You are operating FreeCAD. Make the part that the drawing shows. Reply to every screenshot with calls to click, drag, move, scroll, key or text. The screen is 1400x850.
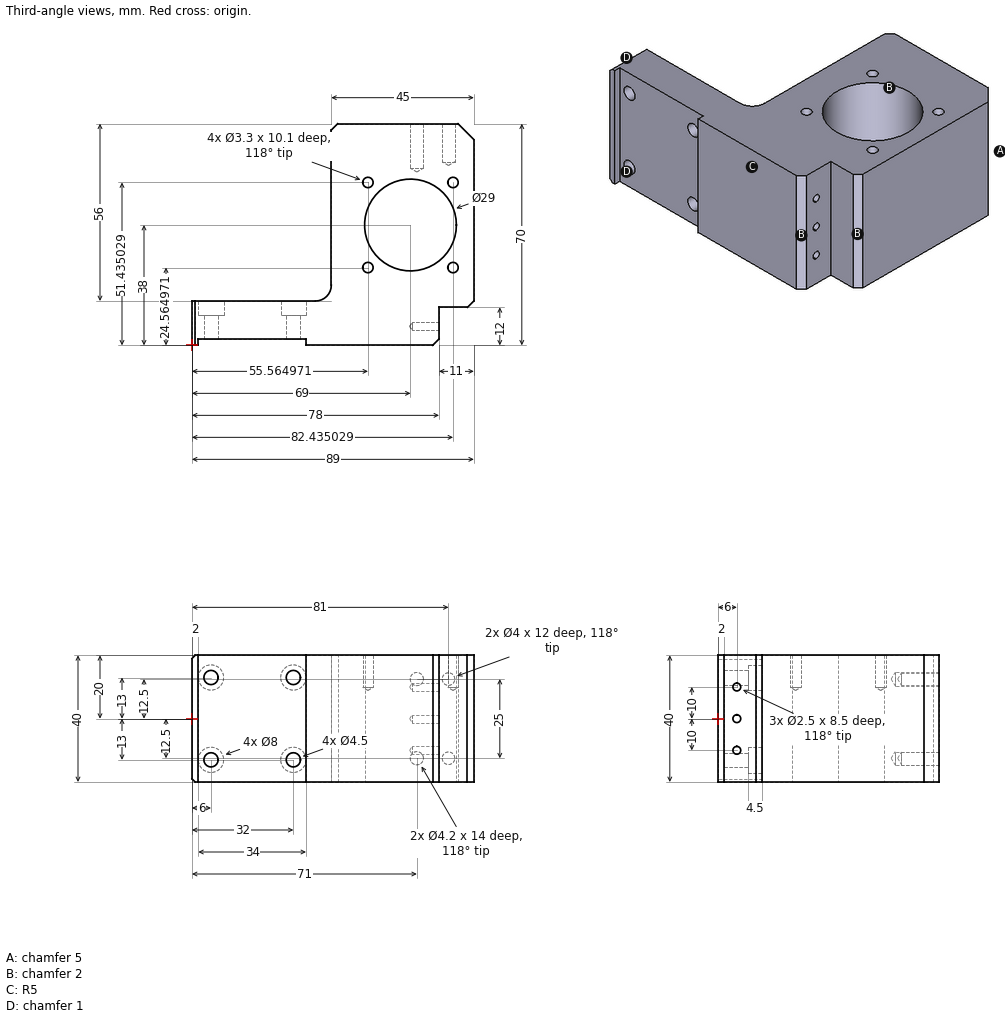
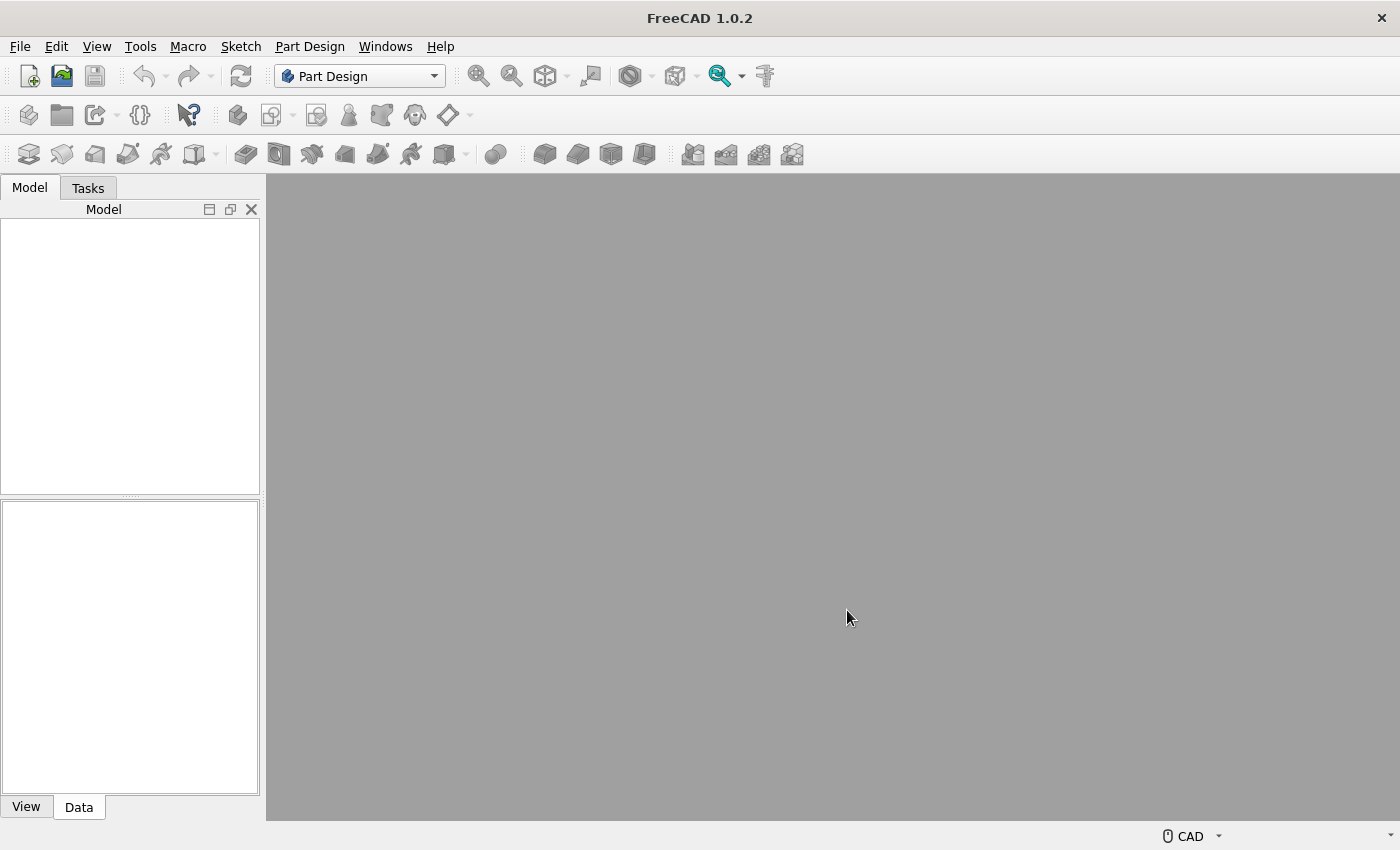
click(29, 76)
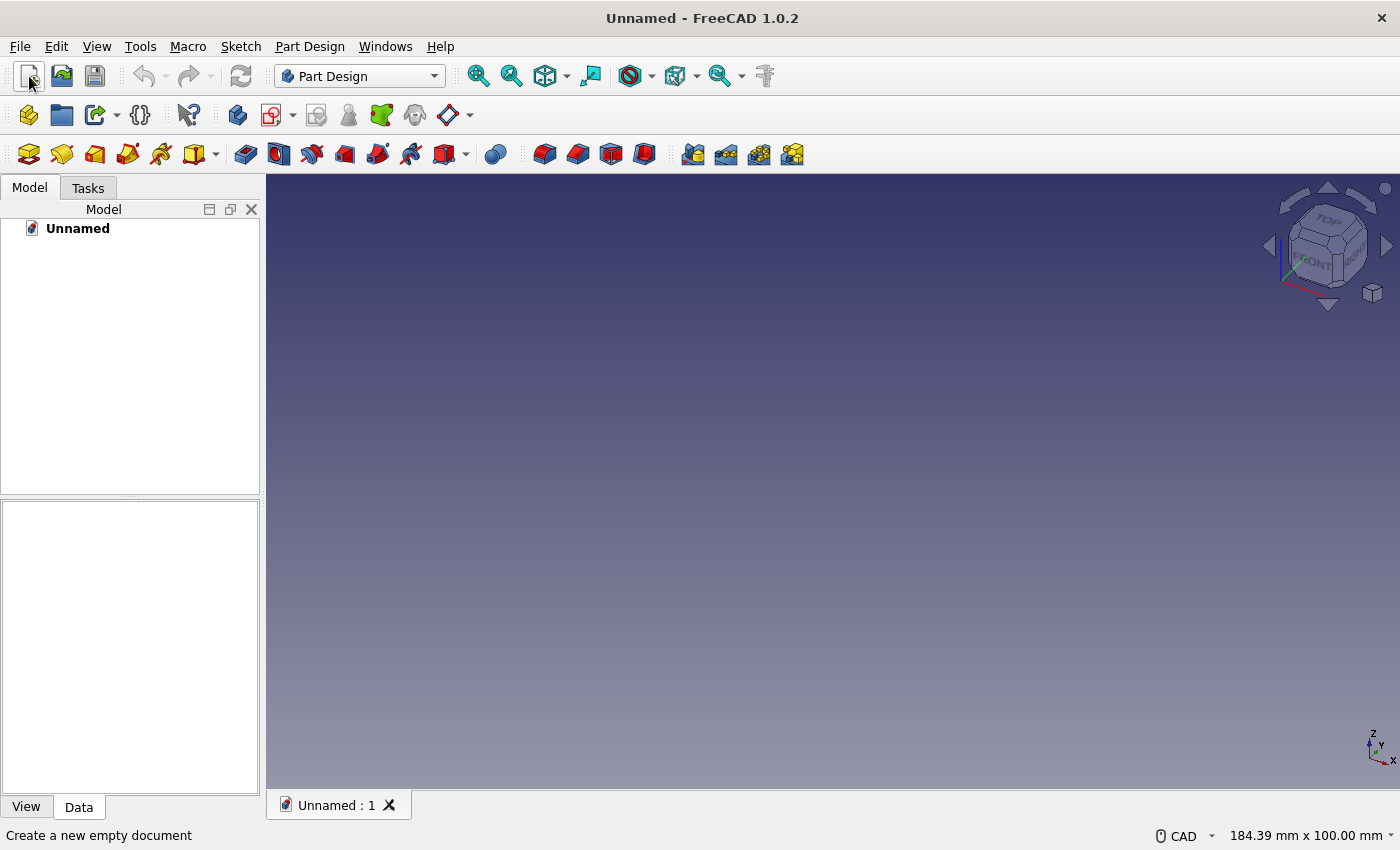
click(270, 116)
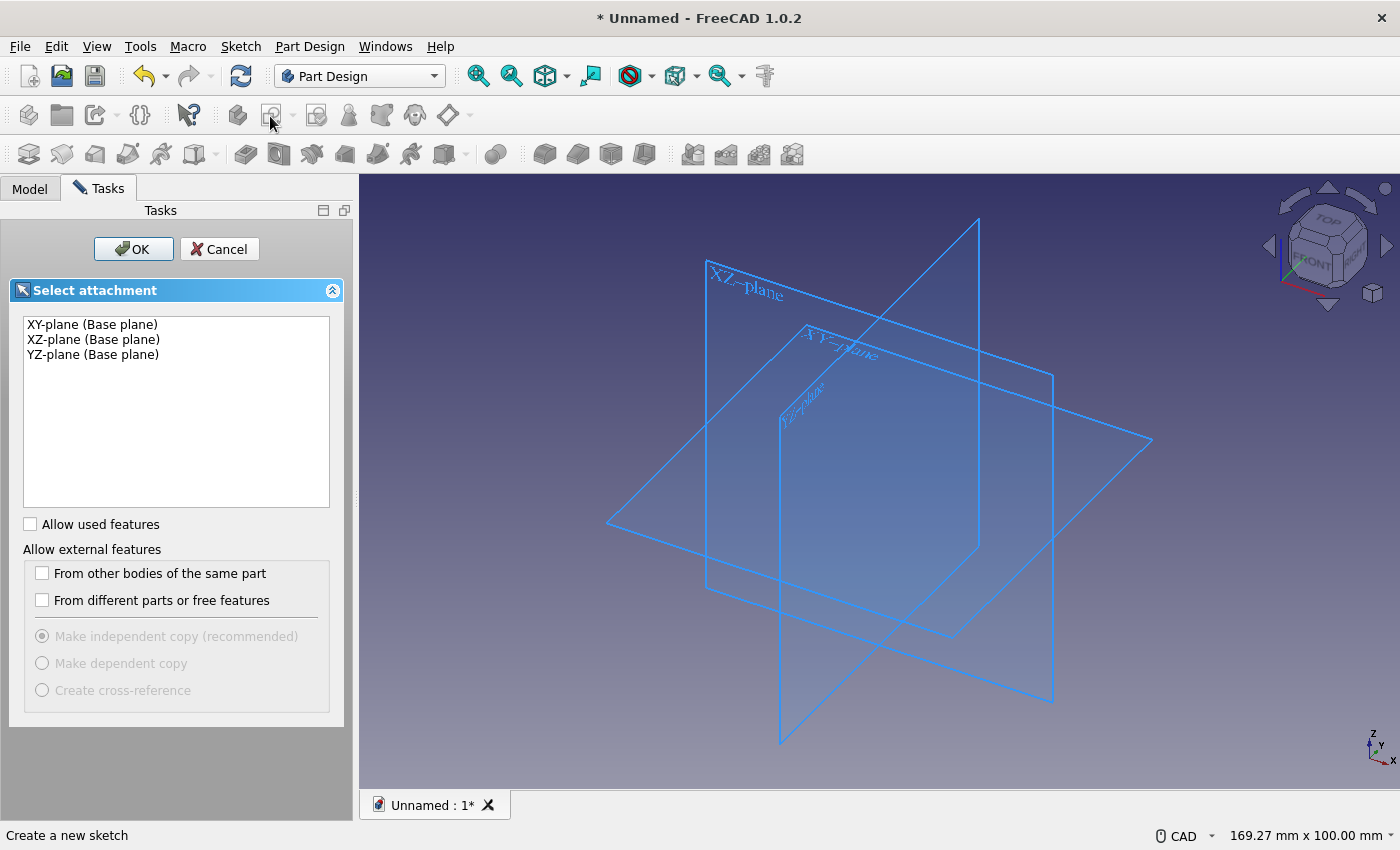
click(84, 324)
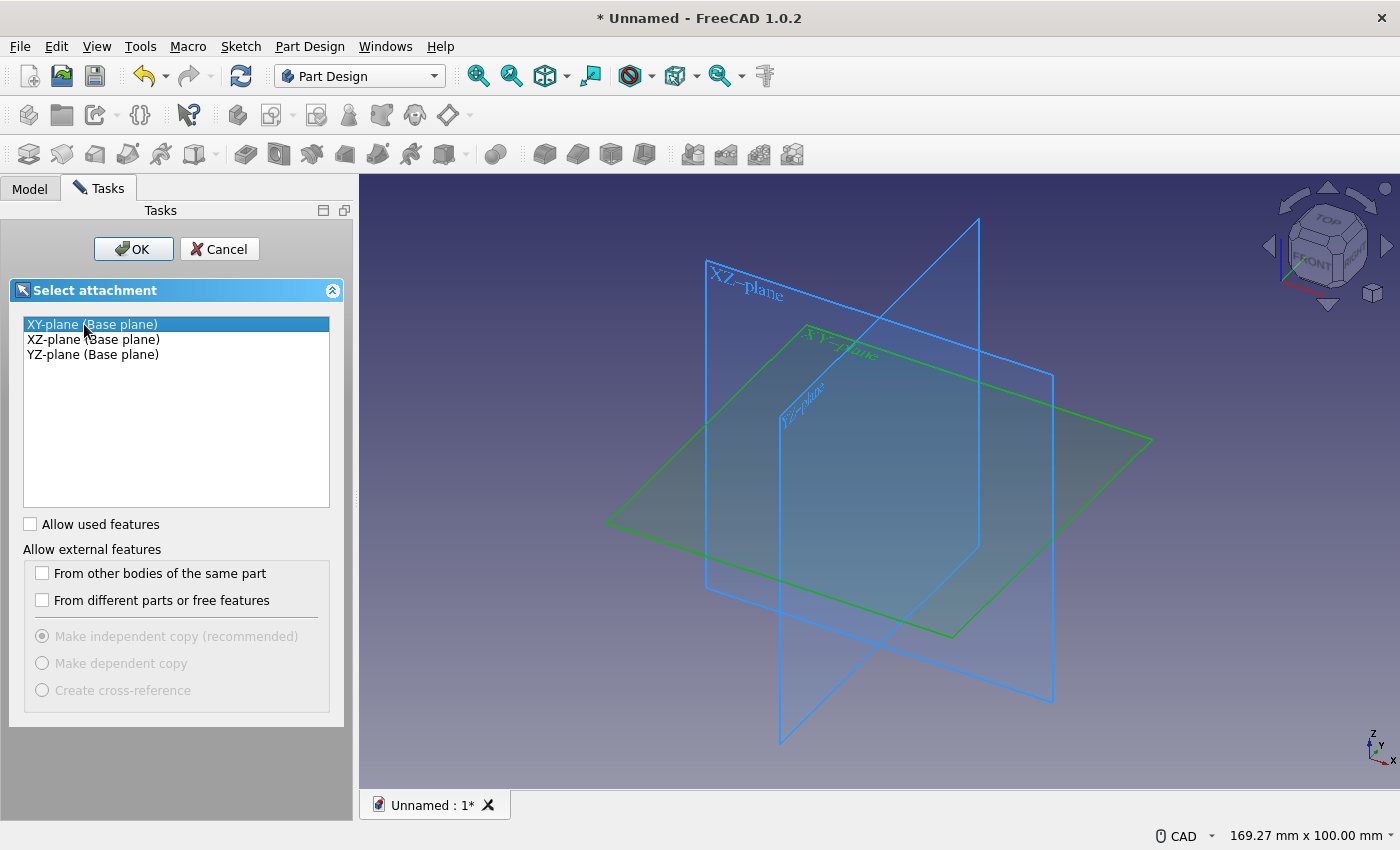
click(134, 249)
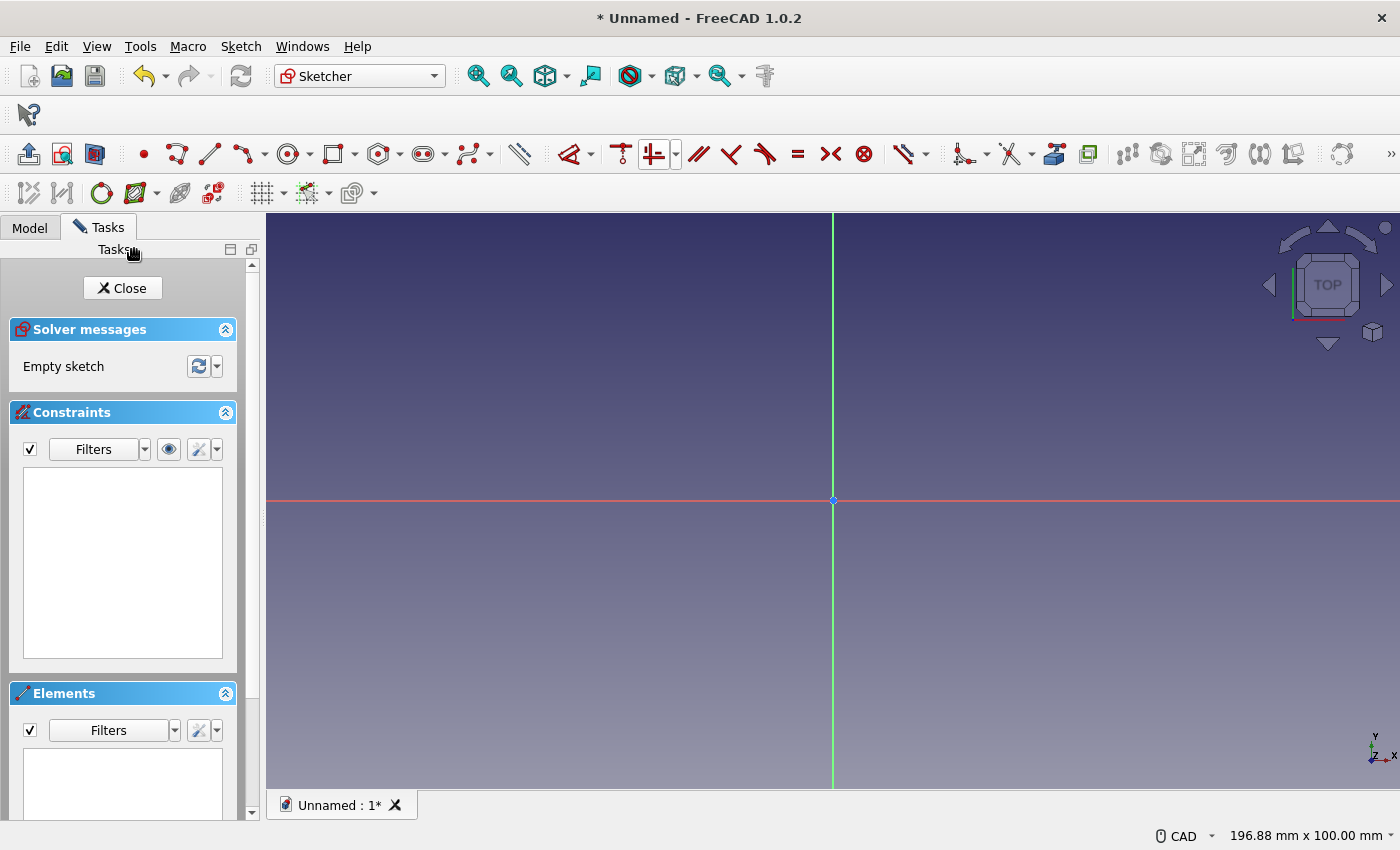
scroll(294, 761, down, 2)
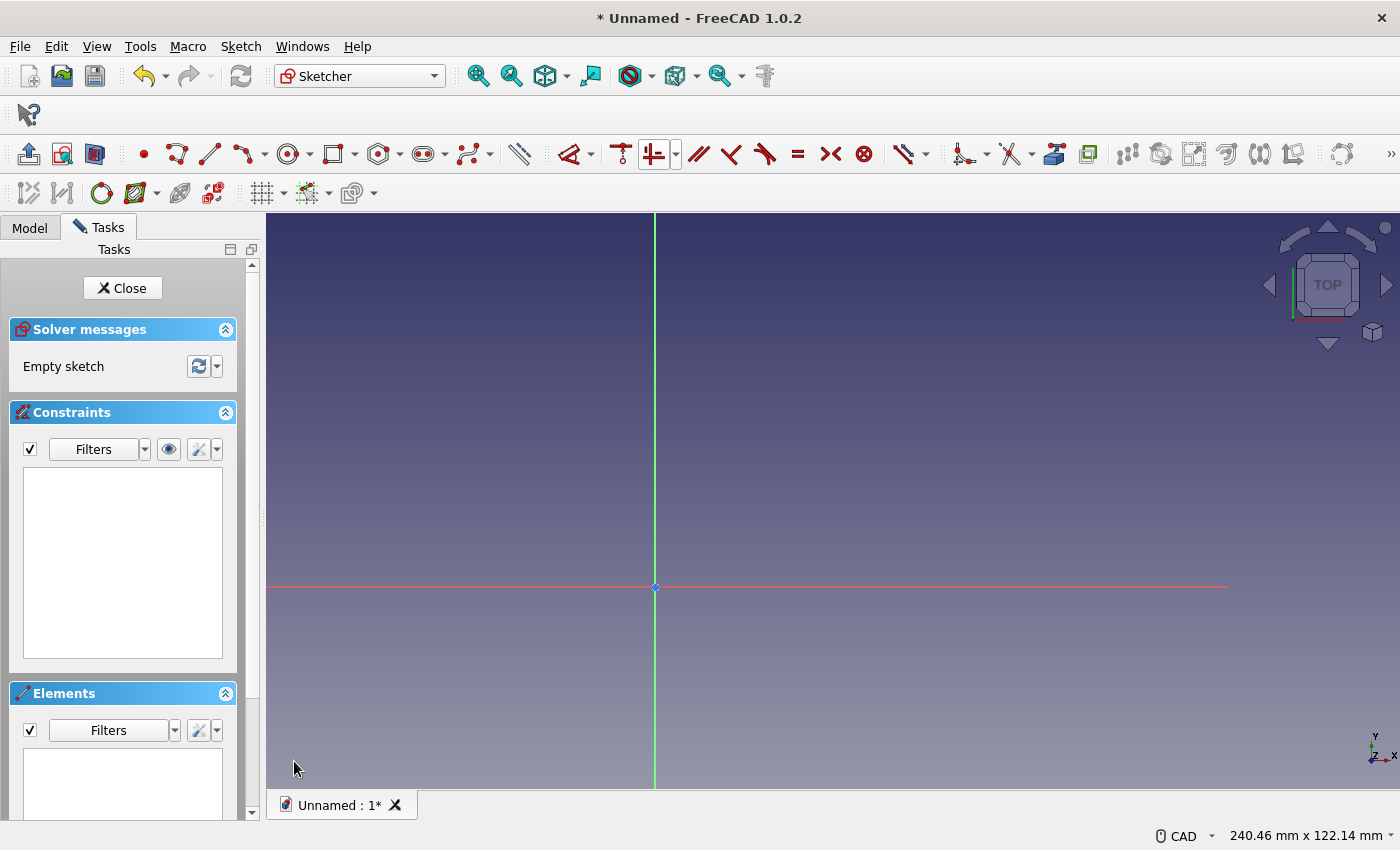
scroll(954, 352, up, 2)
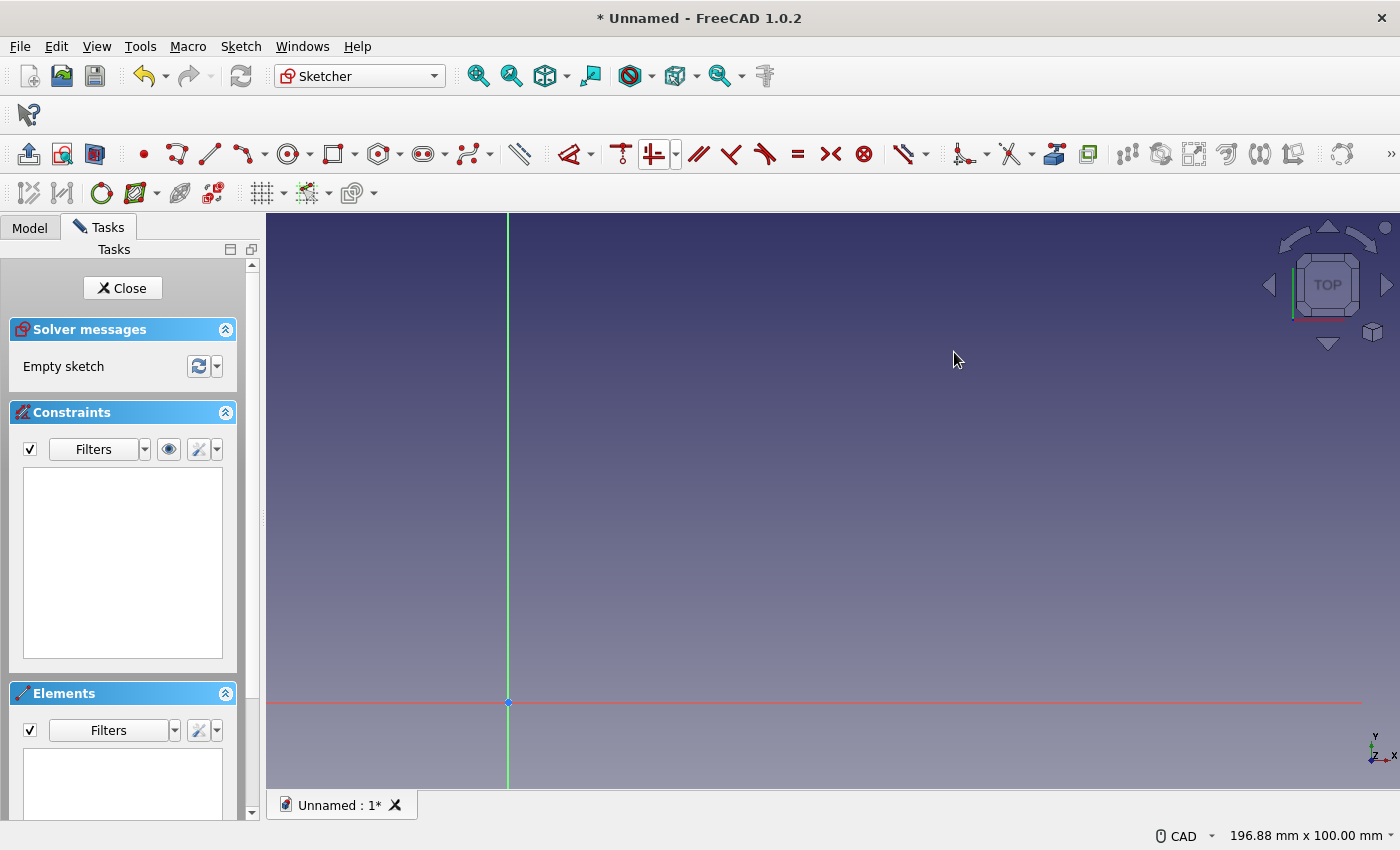
click(177, 154)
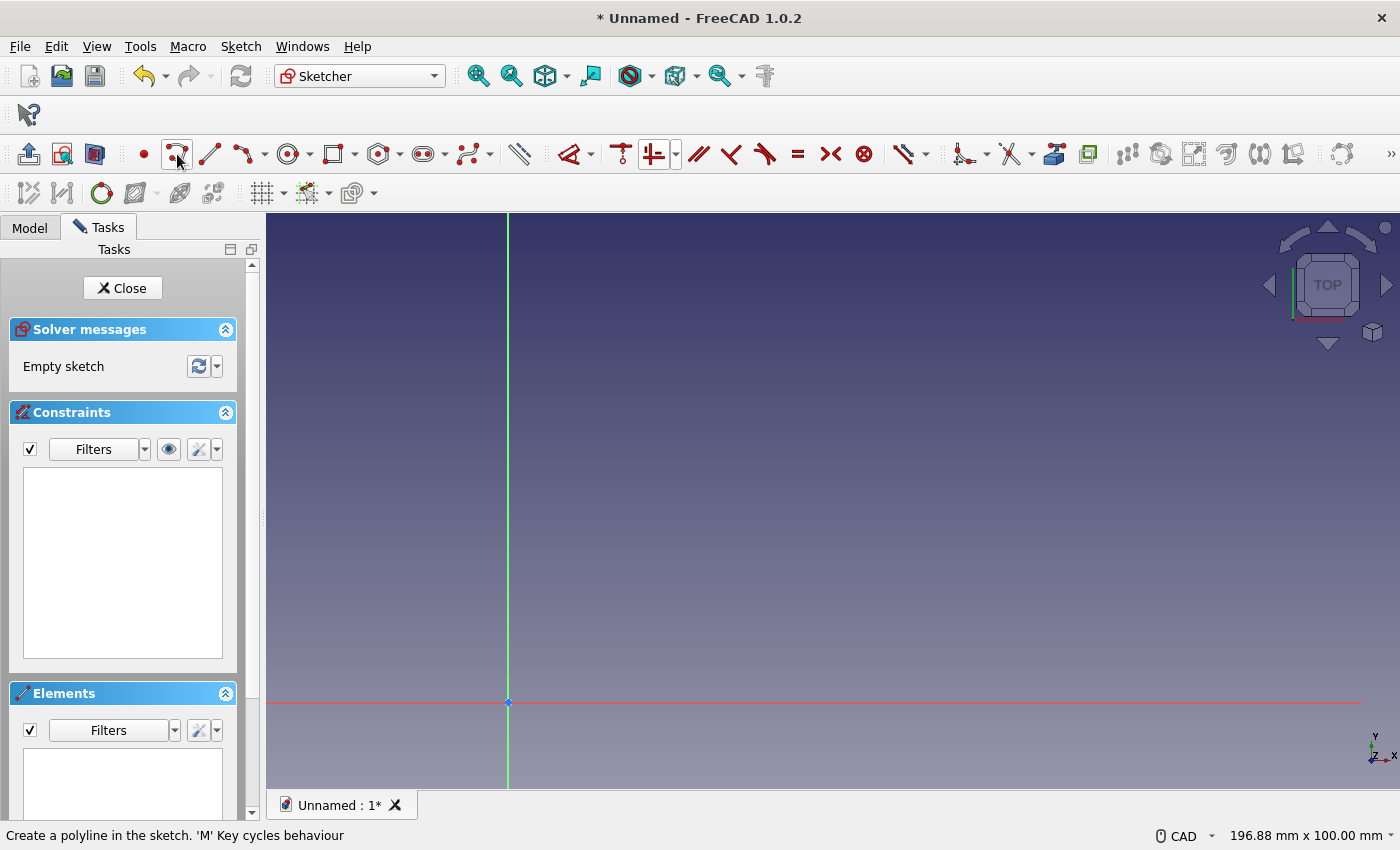
click(508, 703)
click(1021, 694)
click(1021, 299)
click(762, 299)
click(762, 622)
click(517, 622)
click(508, 703)